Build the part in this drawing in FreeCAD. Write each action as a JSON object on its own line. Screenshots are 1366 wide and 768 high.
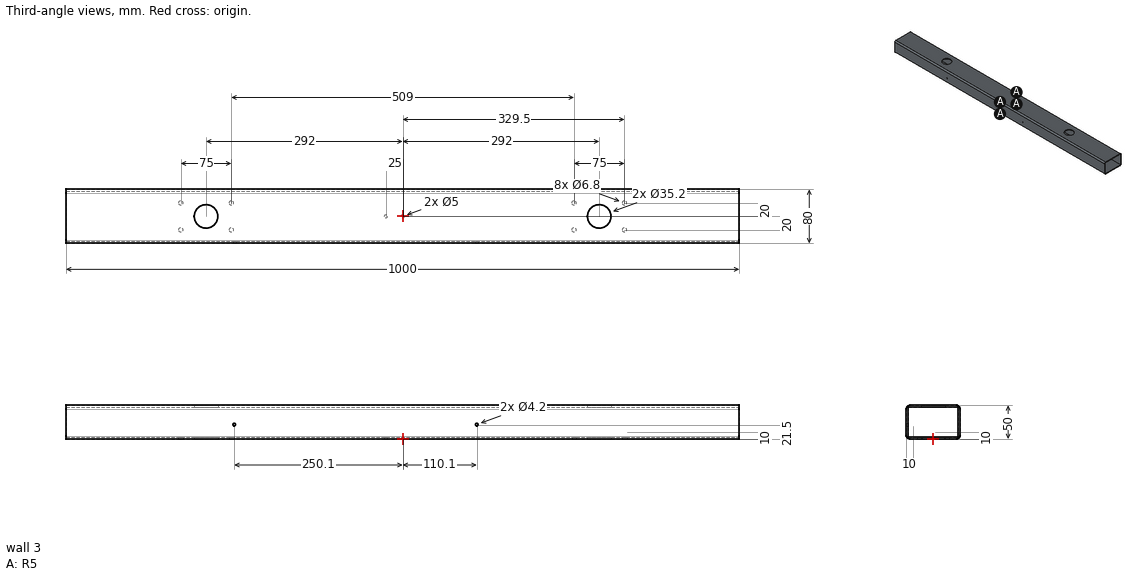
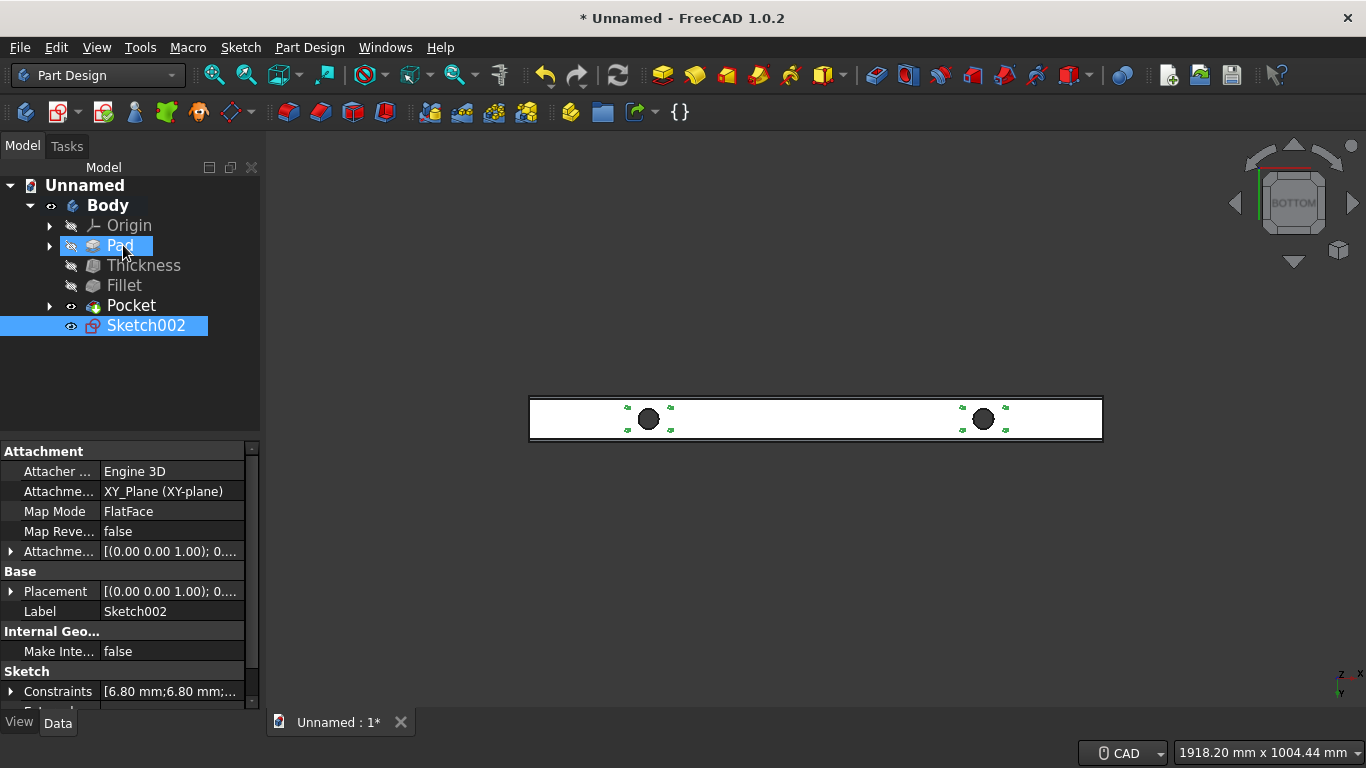
{"action": "left_click", "coordinate": [878, 76]}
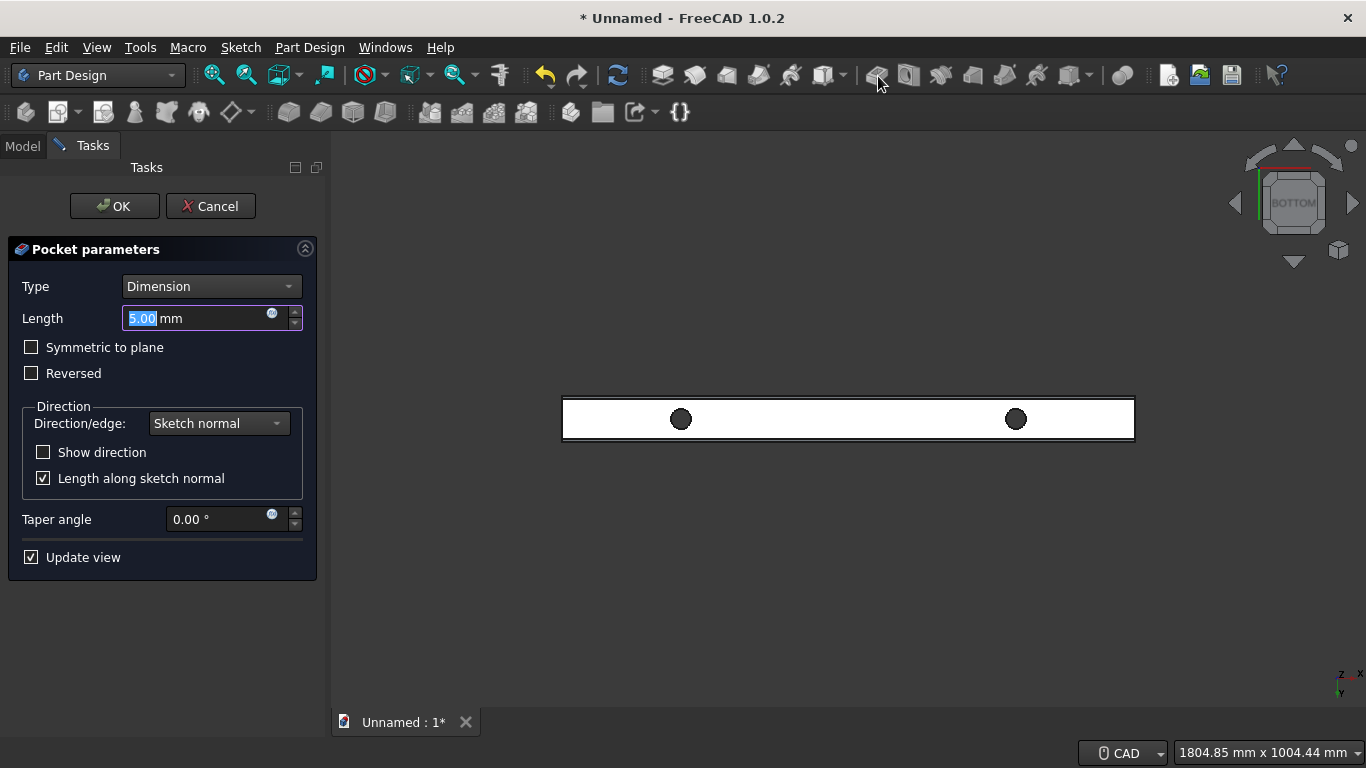
{"action": "type", "text": "10"}
{"action": "key", "text": "Tab"}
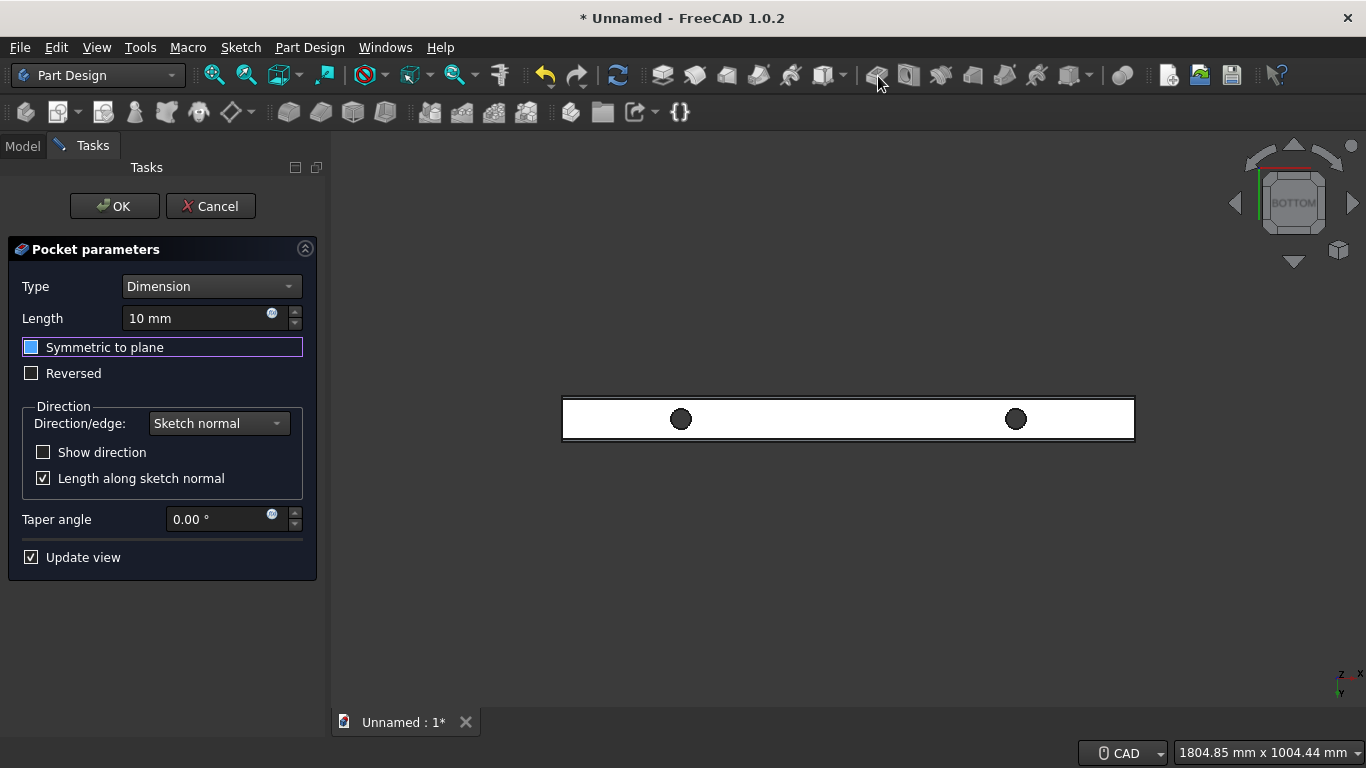
{"action": "left_click", "coordinate": [30, 373]}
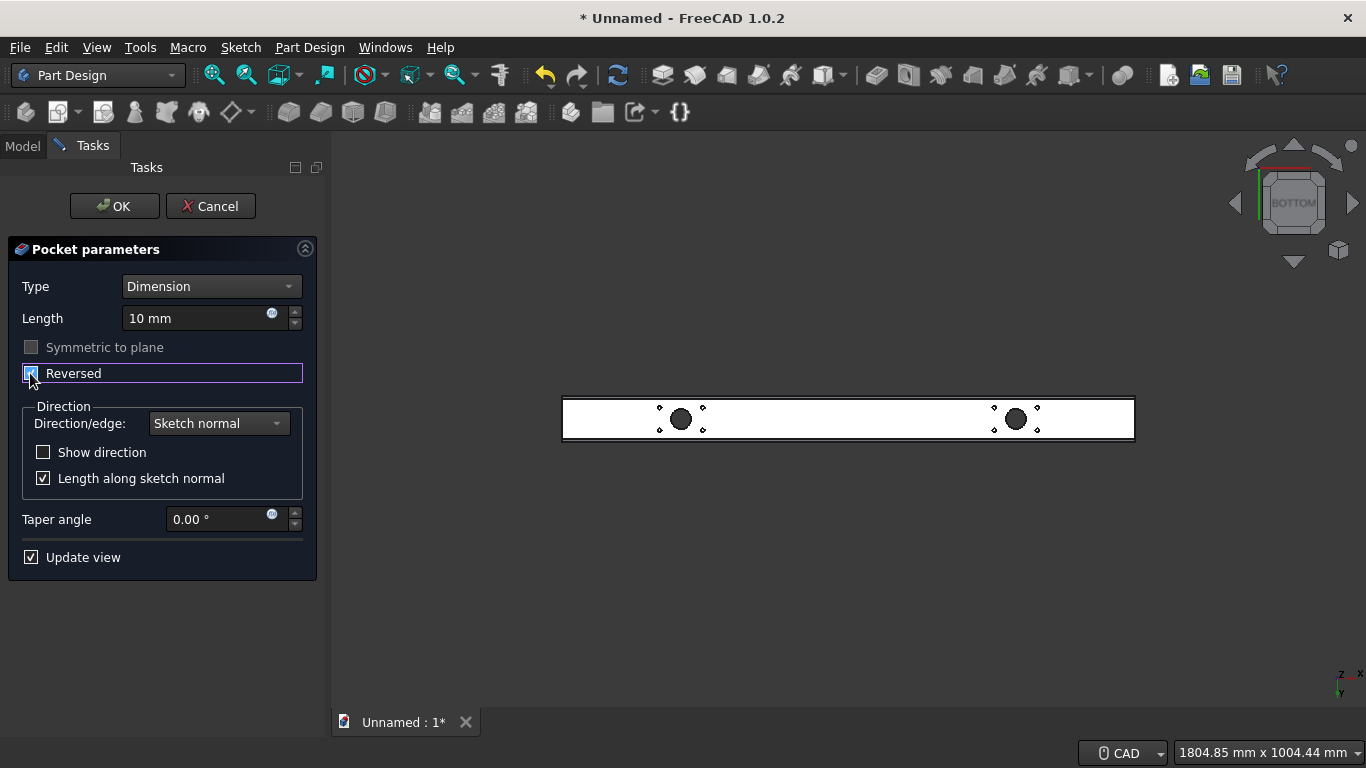
{"action": "left_click", "coordinate": [115, 206]}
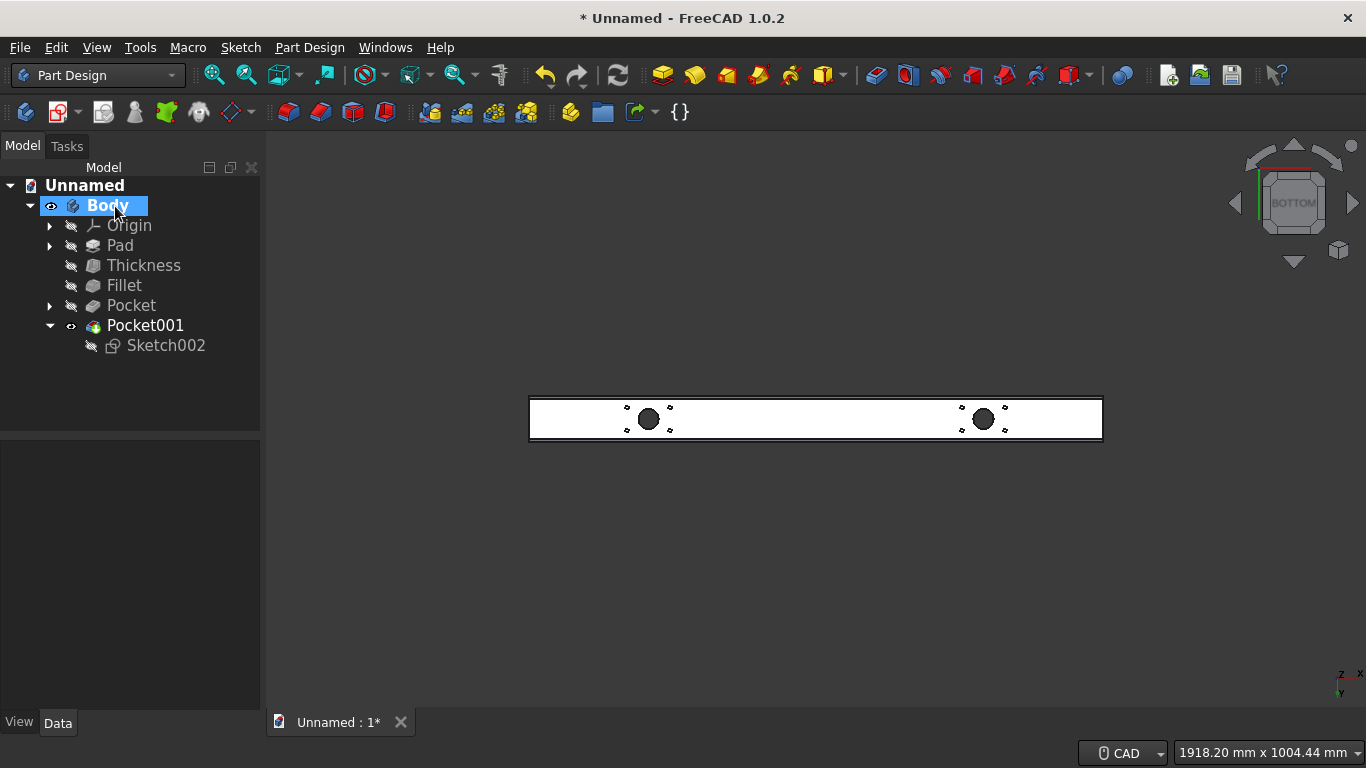
{"action": "left_click", "coordinate": [58, 112]}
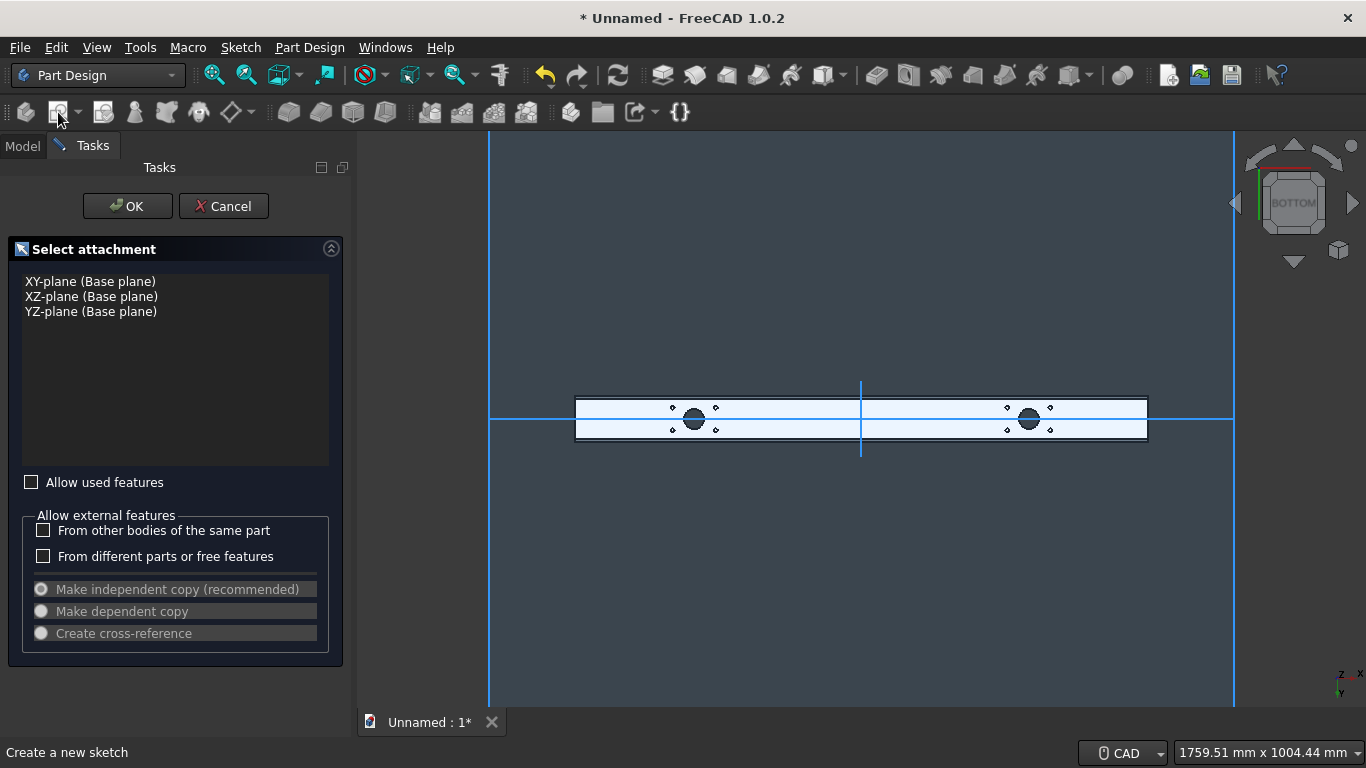
{"action": "left_click", "coordinate": [82, 282]}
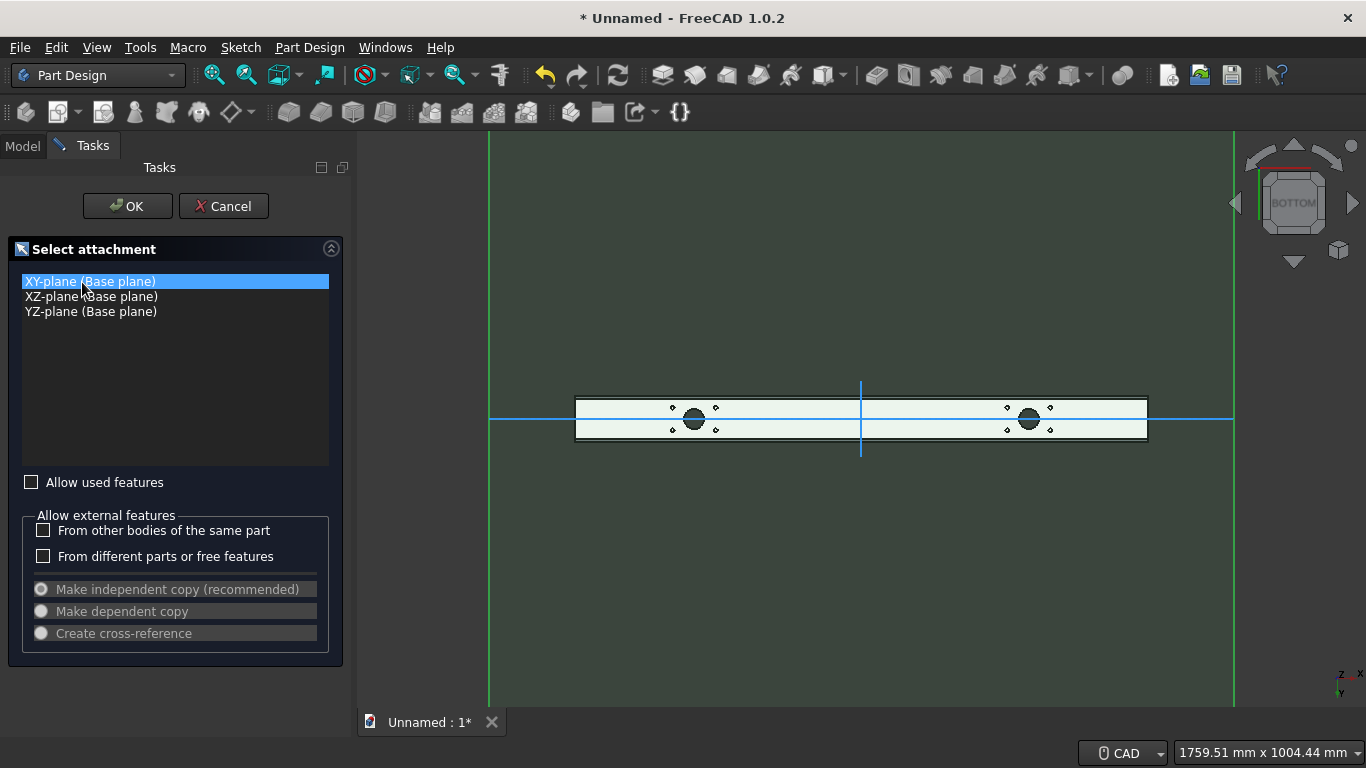
{"action": "left_click", "coordinate": [128, 206]}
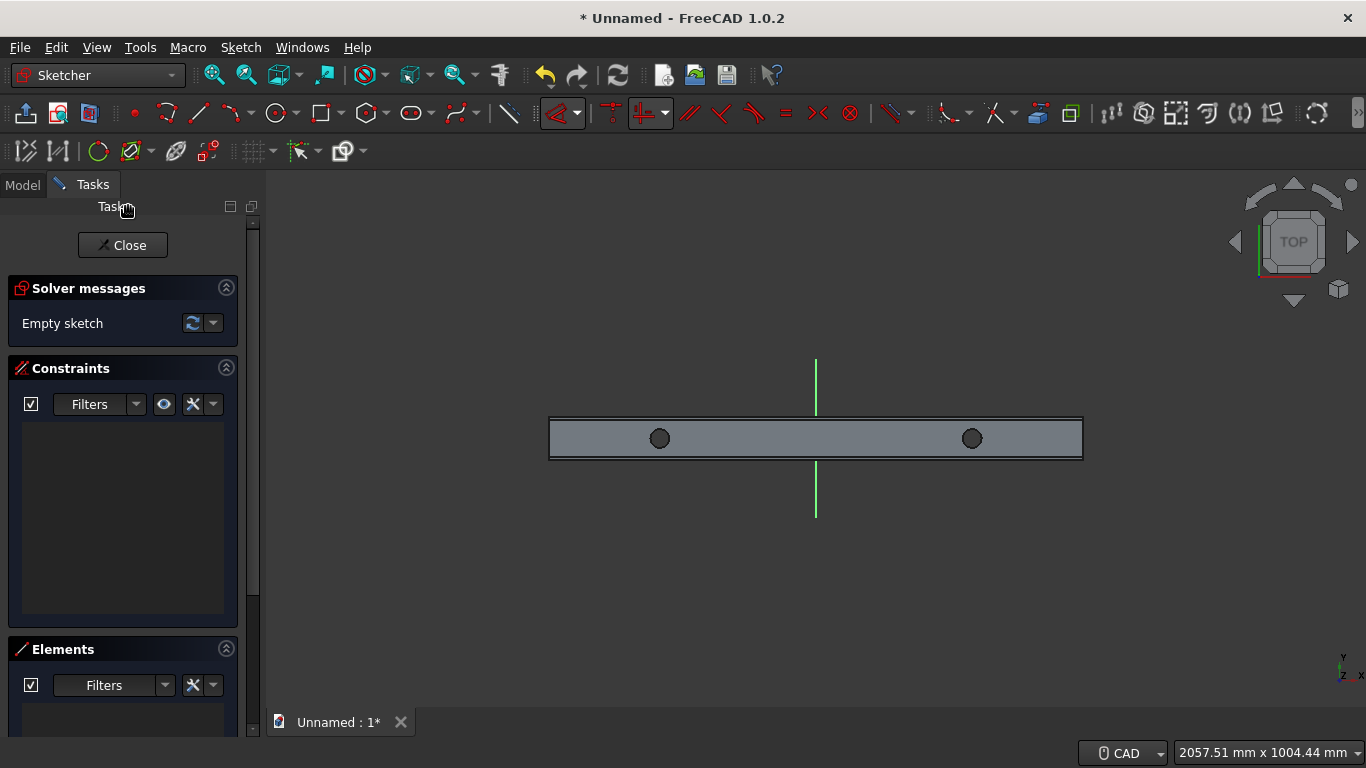
{"action": "left_click", "coordinate": [90, 114]}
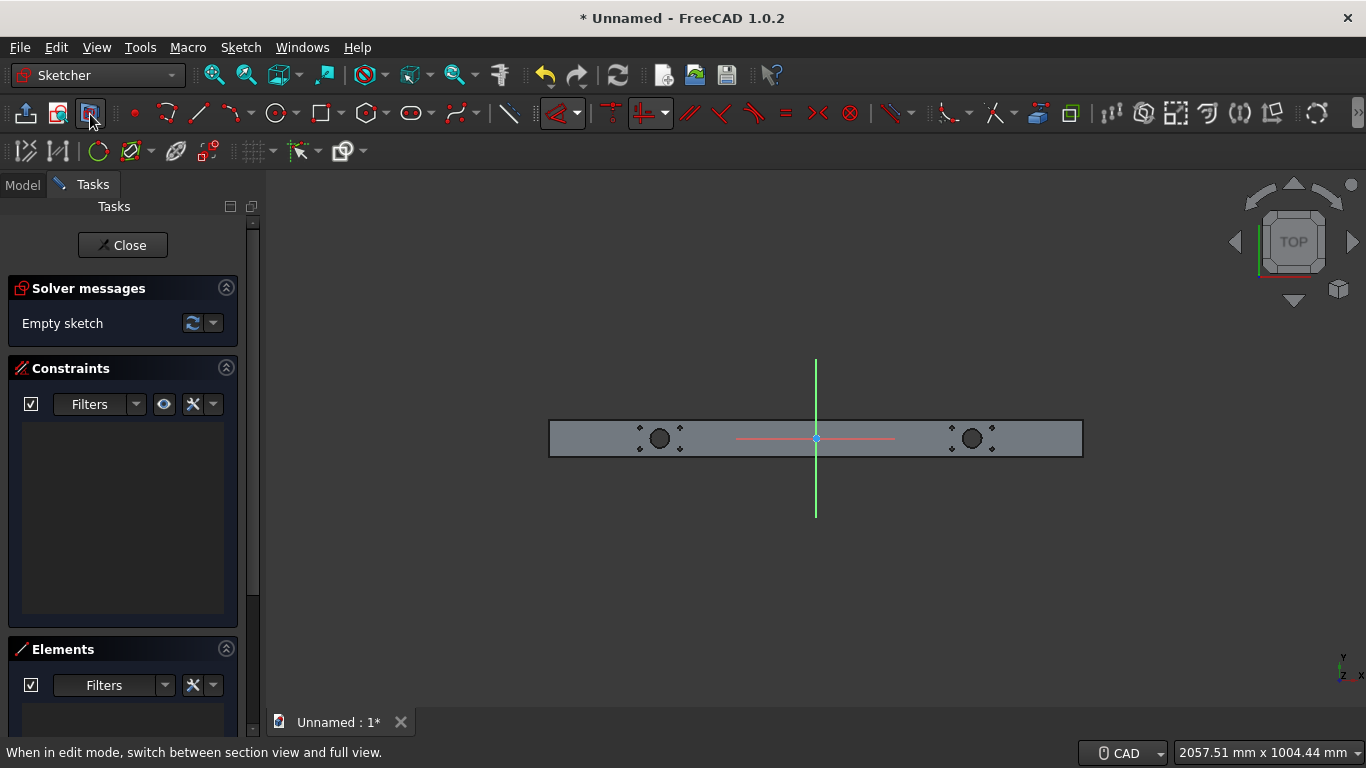
{"action": "scroll", "coordinate": [813, 438], "scroll_direction": "up", "scroll_amount": 15}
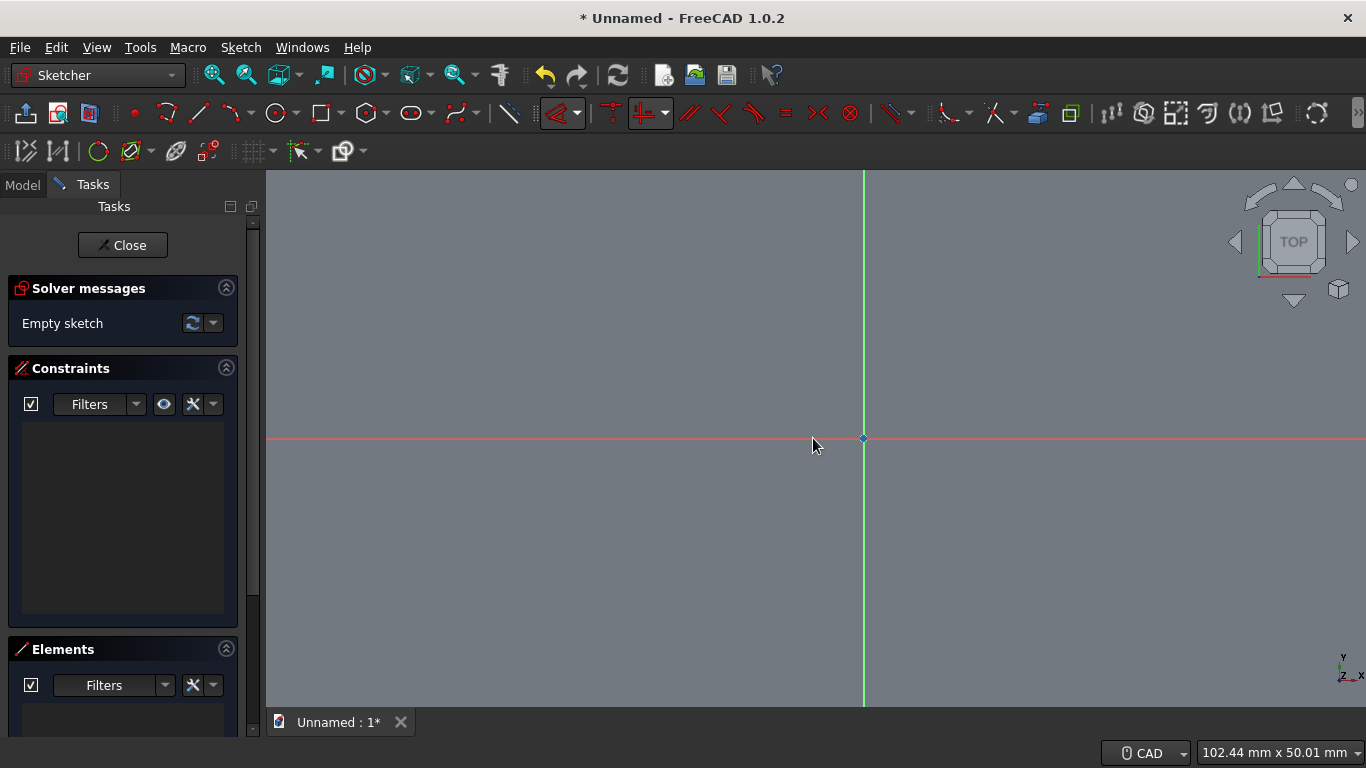
{"action": "scroll", "coordinate": [708, 438], "scroll_direction": "up", "scroll_amount": 3}